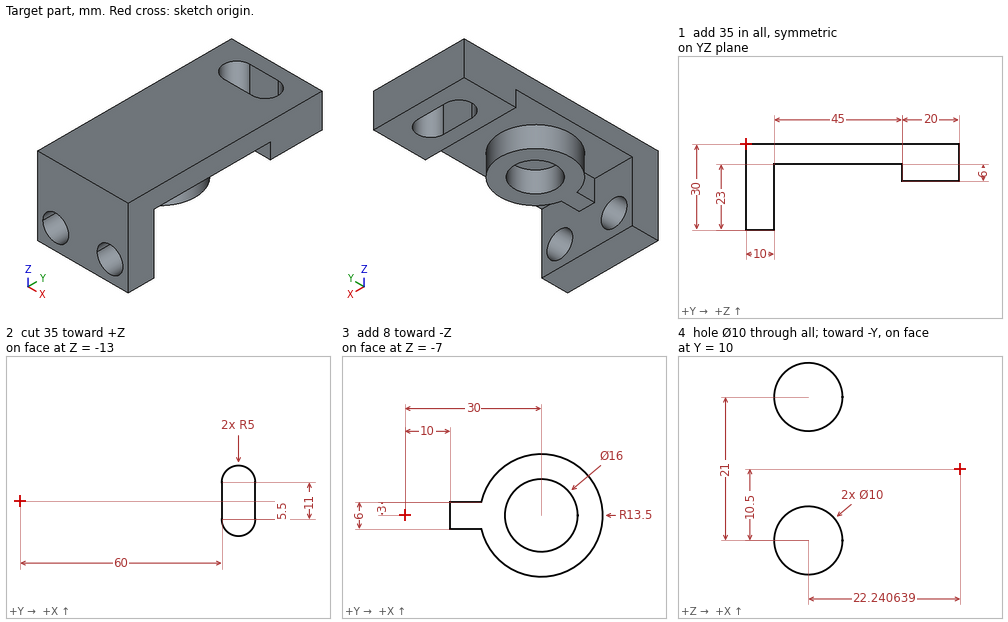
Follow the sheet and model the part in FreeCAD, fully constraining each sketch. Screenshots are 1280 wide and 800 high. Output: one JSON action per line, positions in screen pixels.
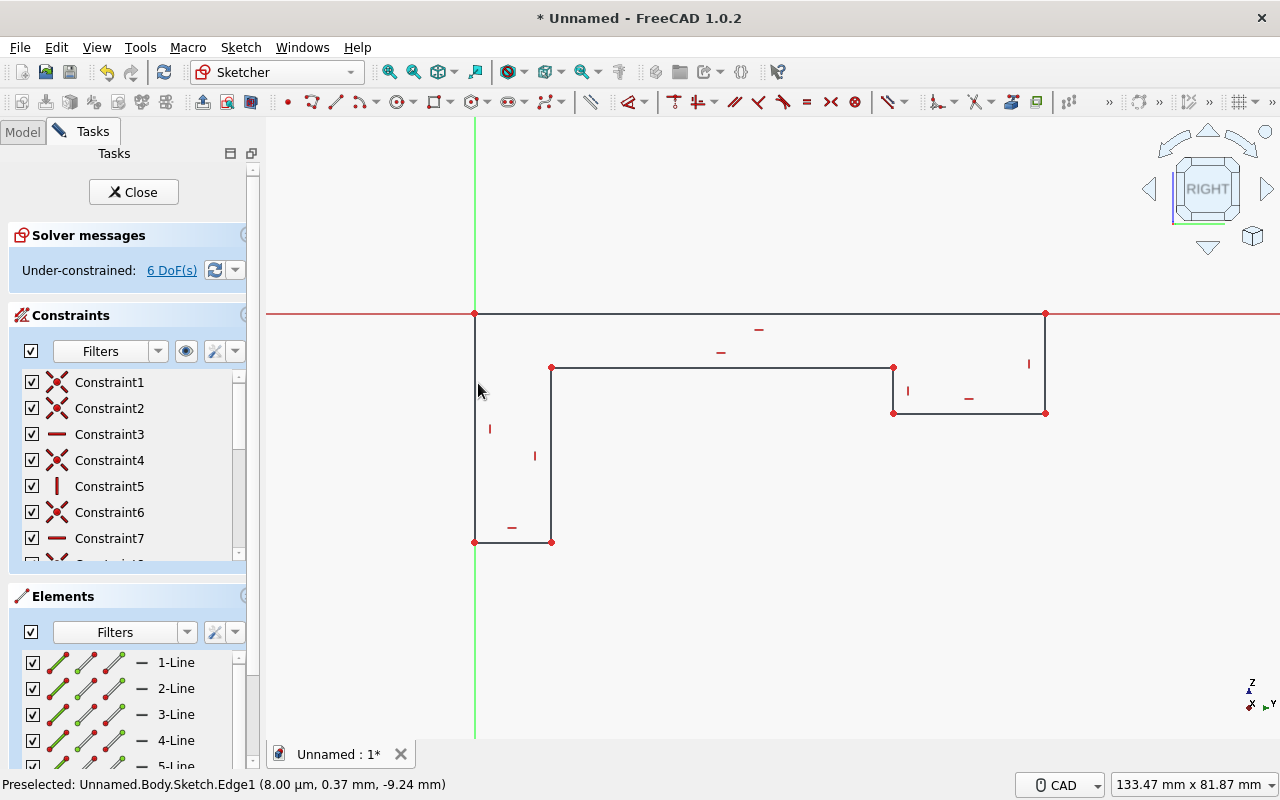
{"action": "left_click", "coordinate": [893, 382]}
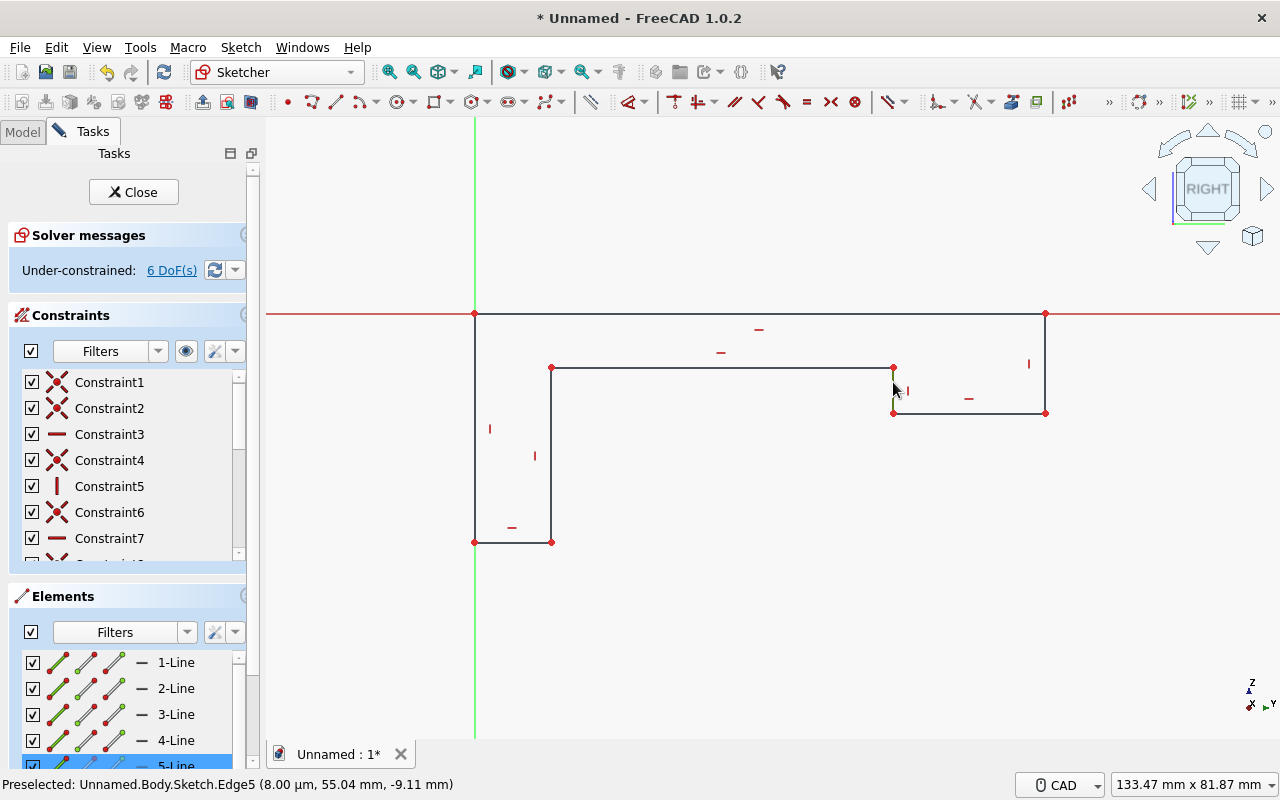
{"action": "left_click", "coordinate": [646, 102]}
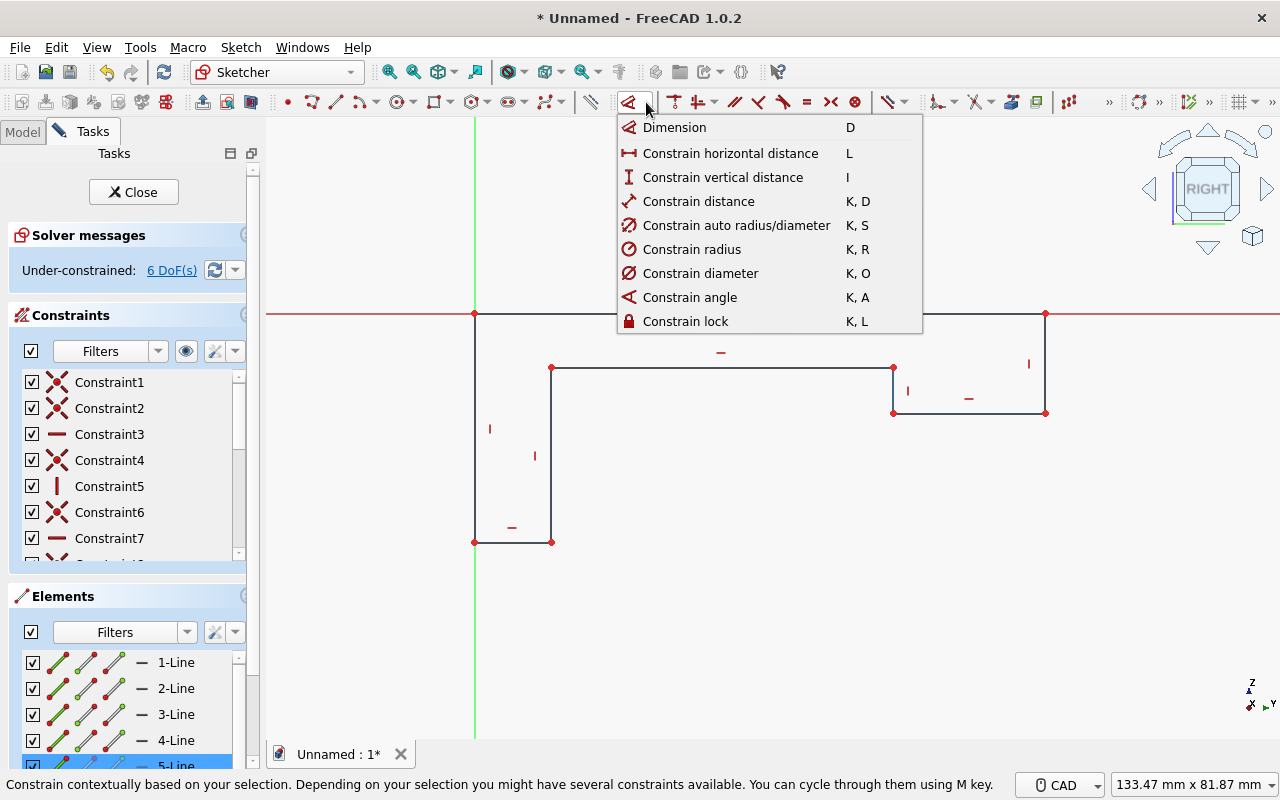
{"action": "left_click", "coordinate": [770, 177]}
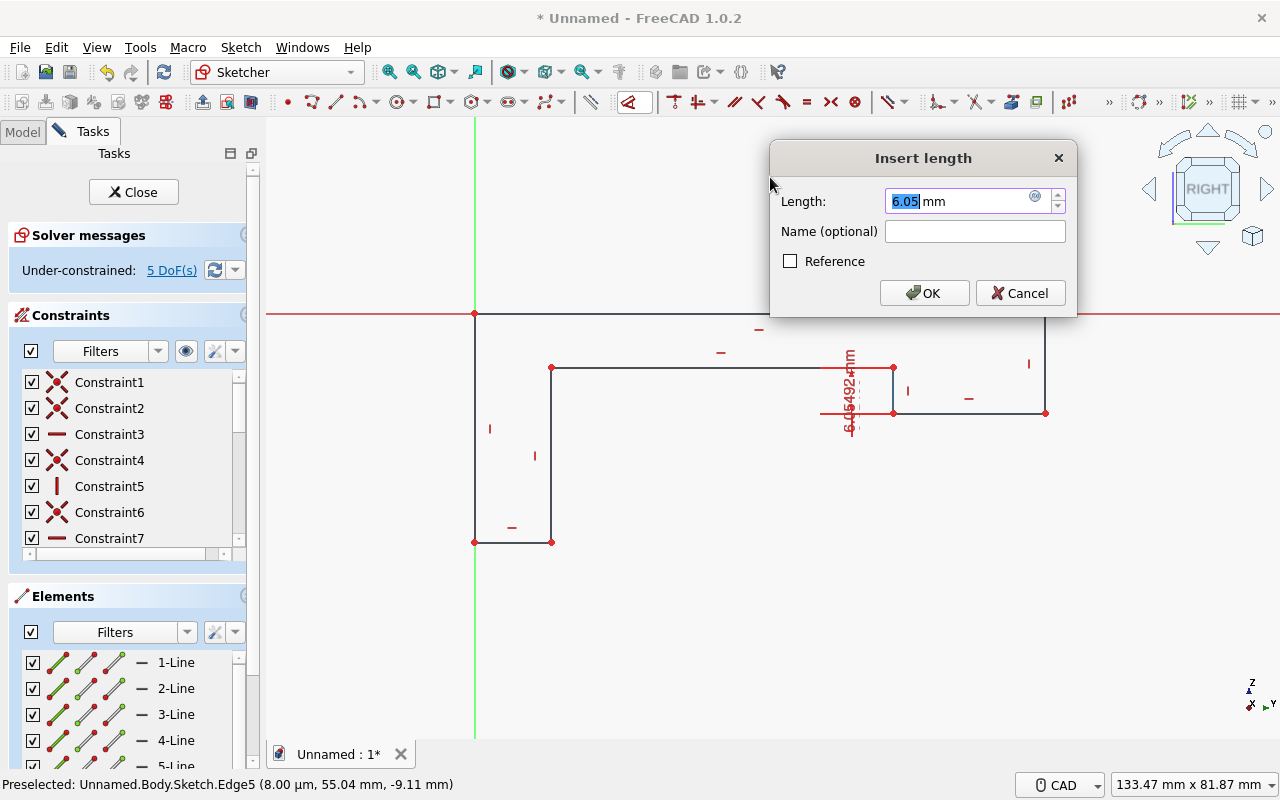
{"action": "type", "text": "6"}
{"action": "key", "text": "Return"}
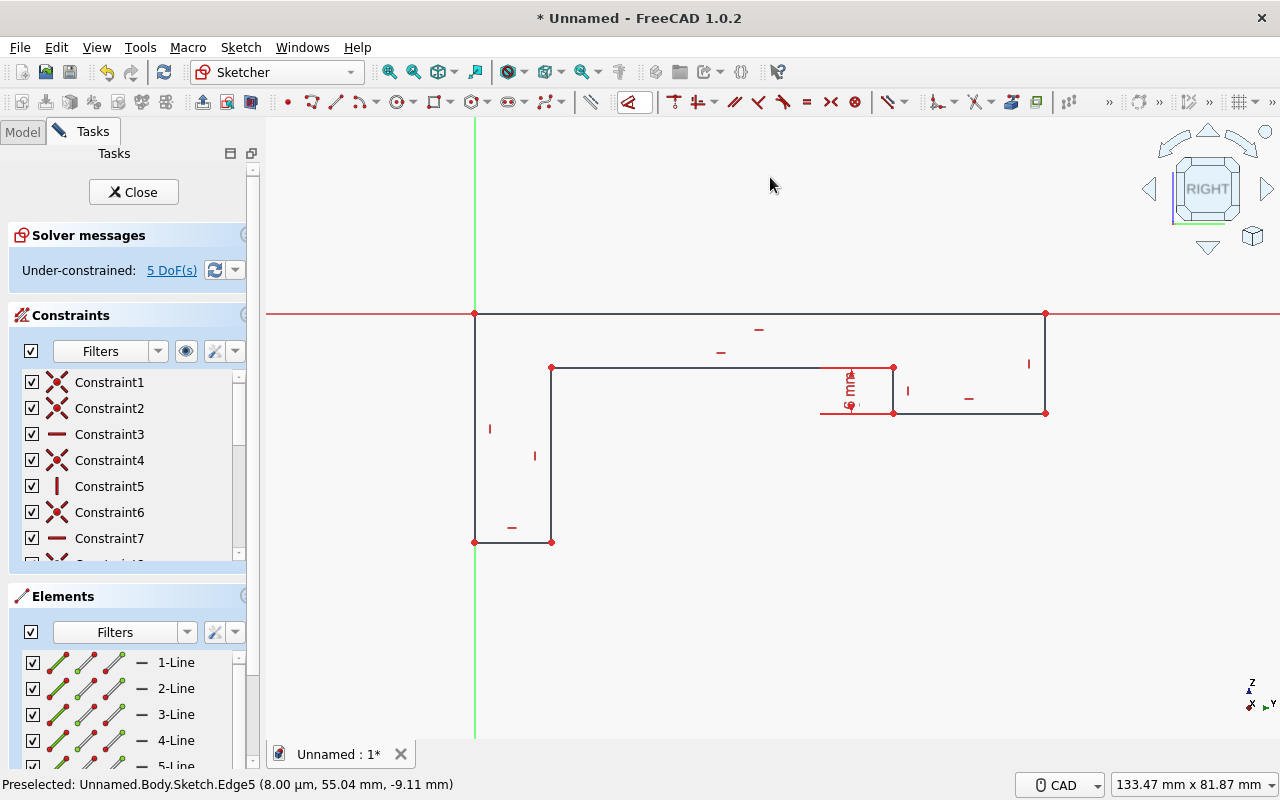
{"action": "left_click", "coordinate": [475, 383]}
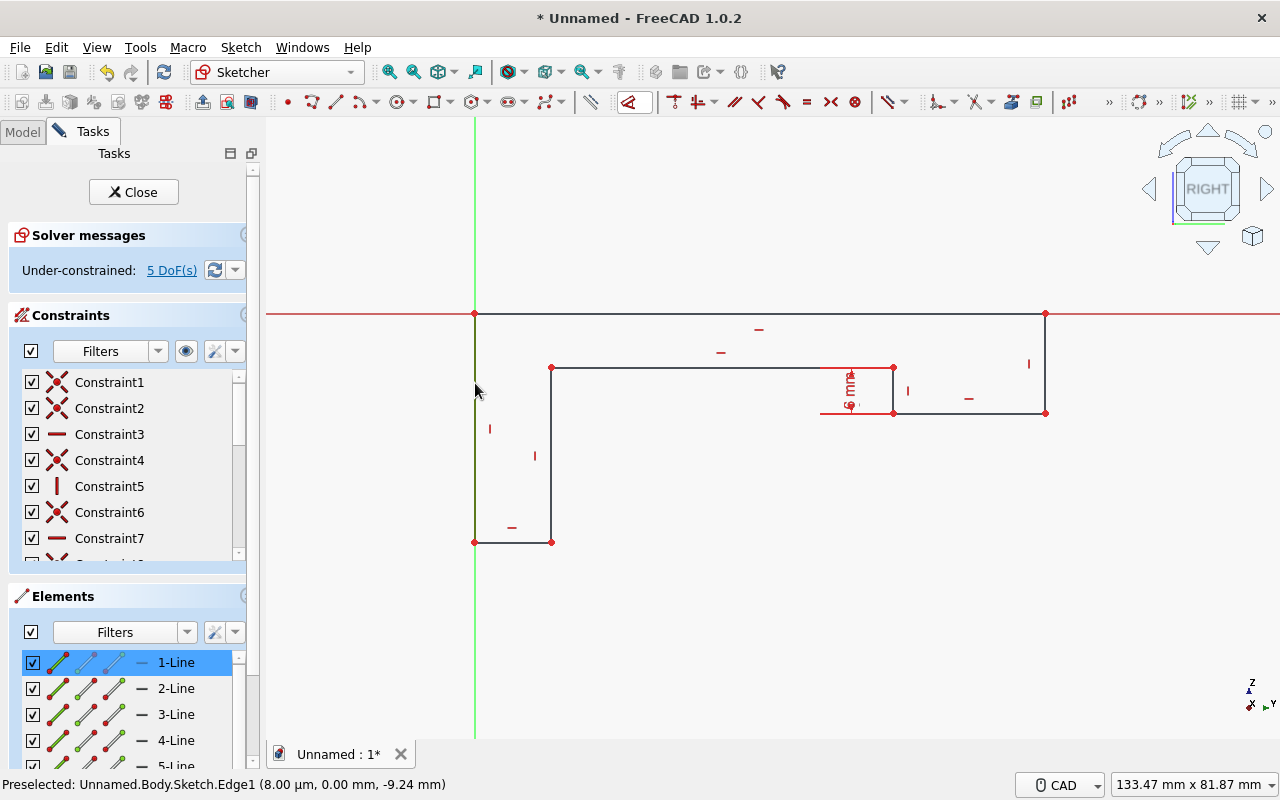
{"action": "left_click", "coordinate": [646, 102]}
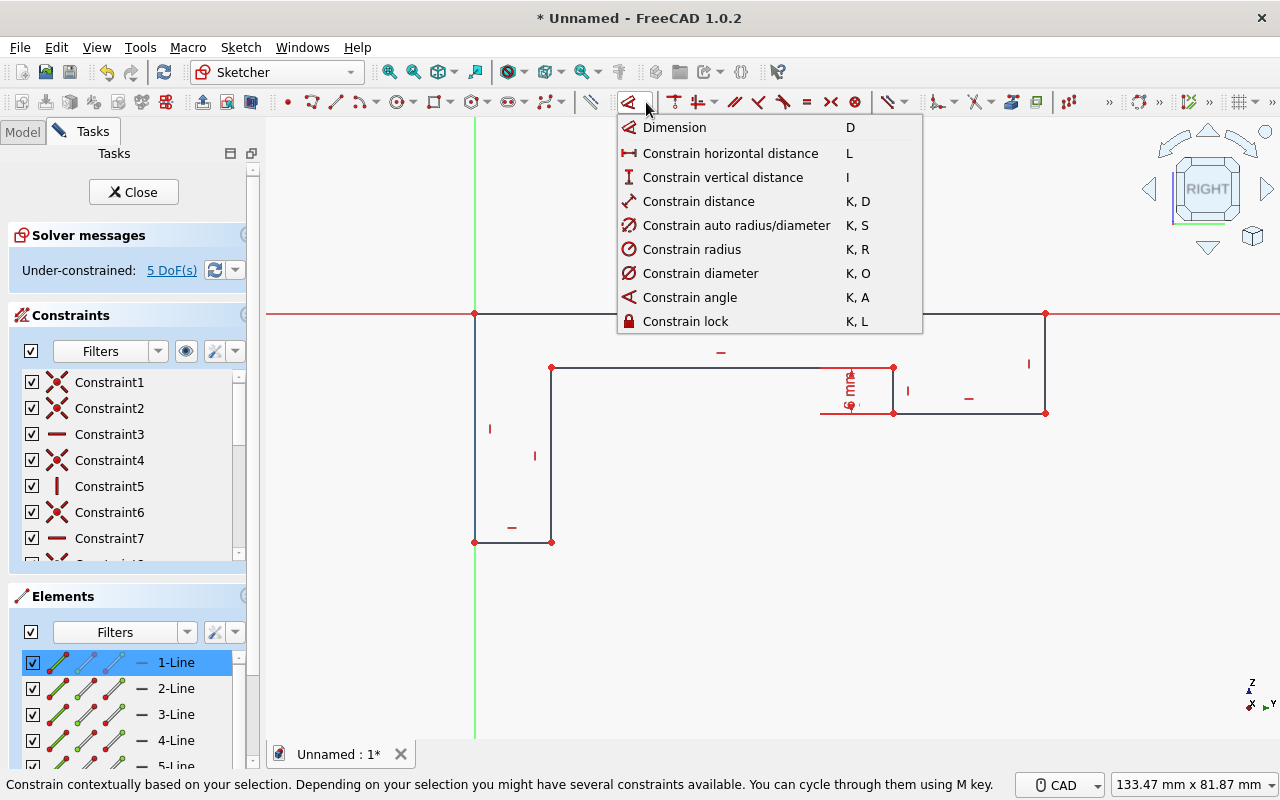
{"action": "left_click", "coordinate": [770, 177]}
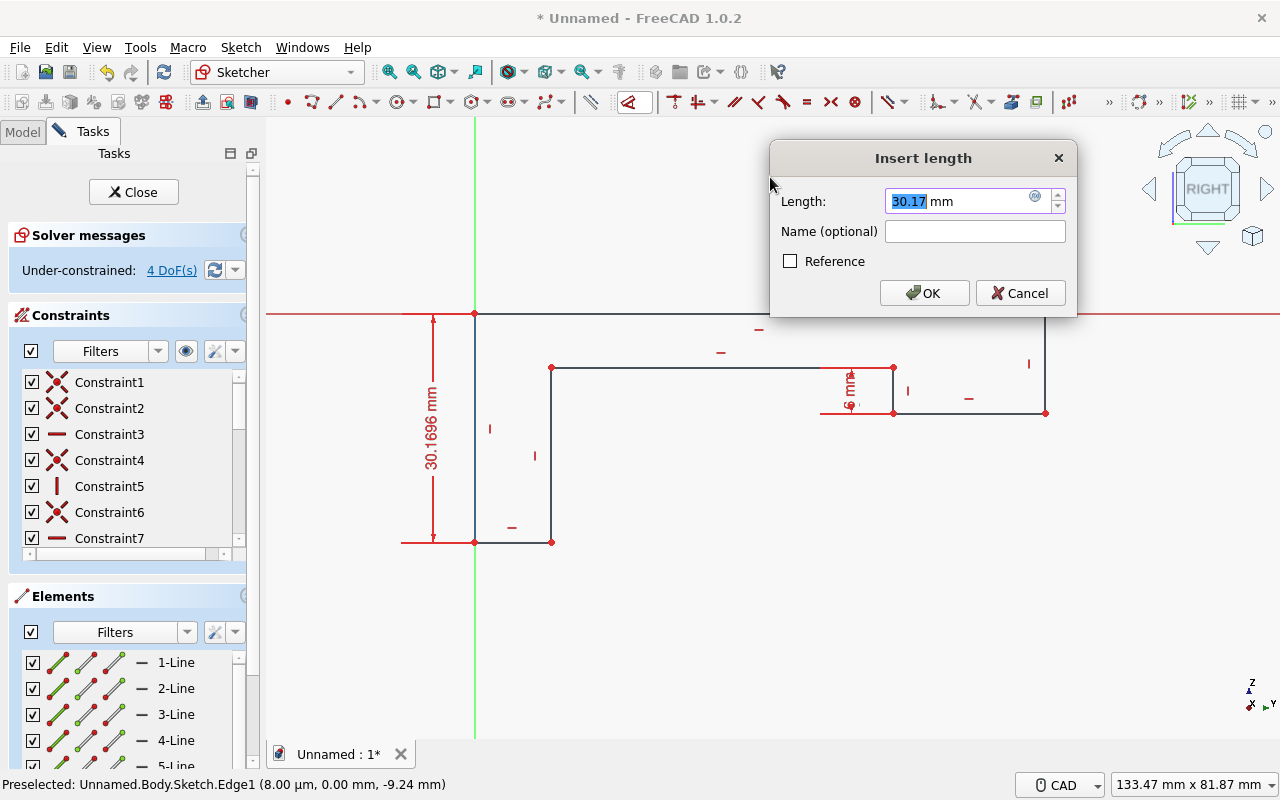
{"action": "type", "text": "30"}
{"action": "key", "text": "Return"}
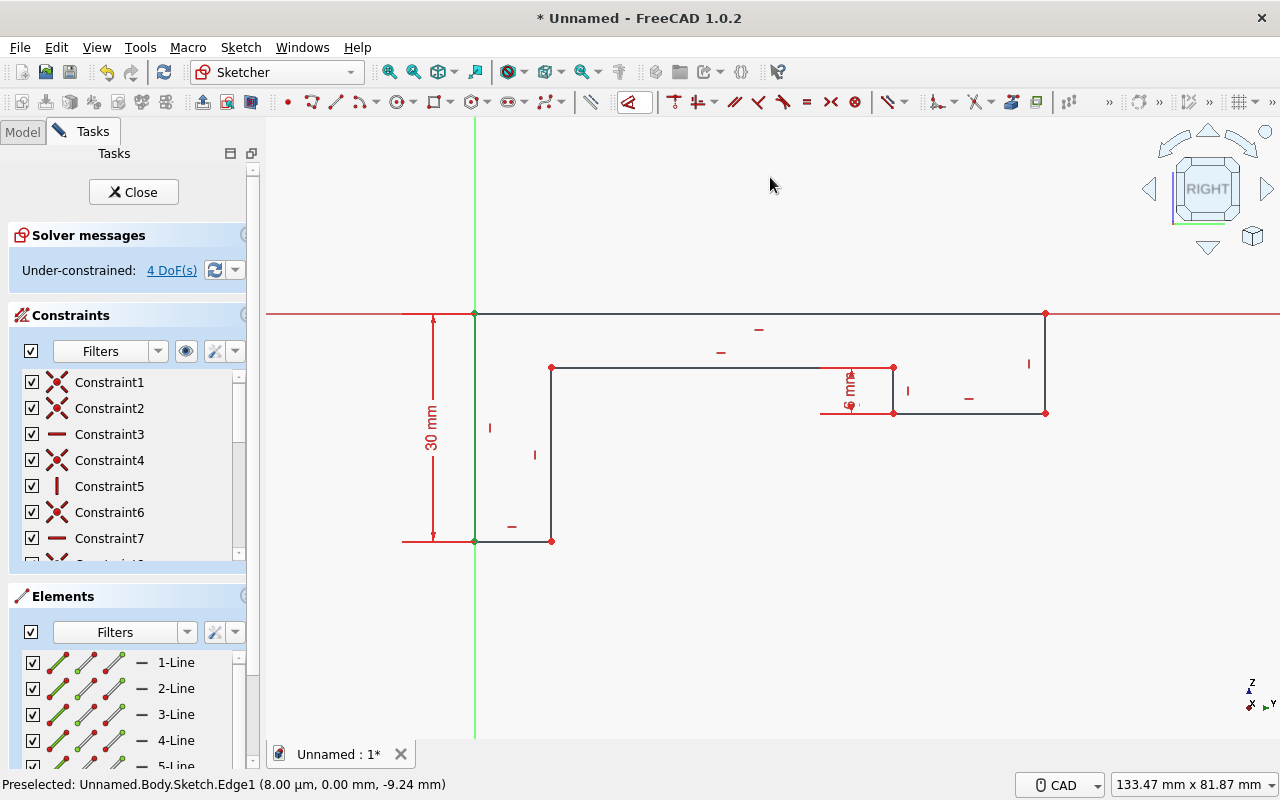
{"action": "left_click", "coordinate": [498, 542]}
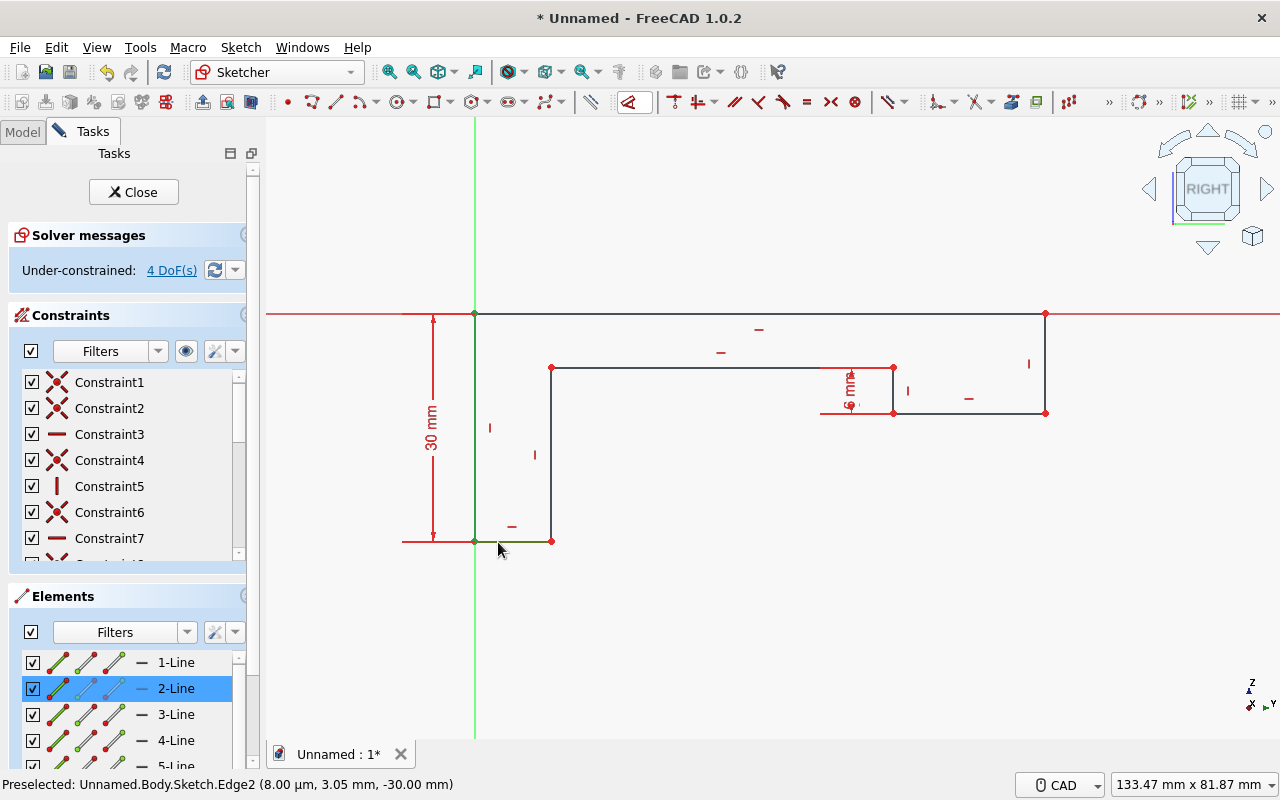
{"action": "key", "text": "l"}